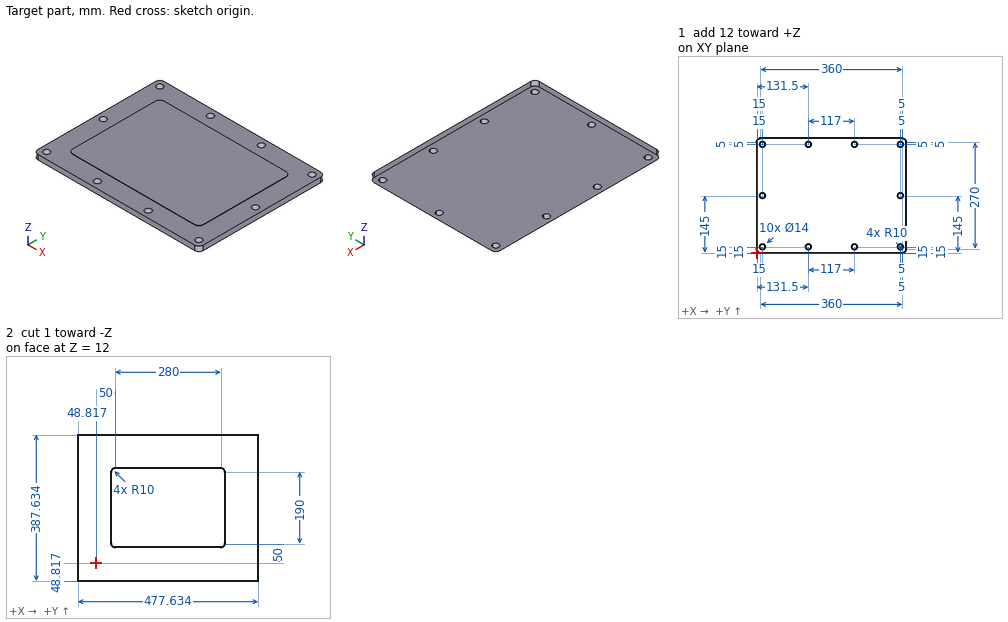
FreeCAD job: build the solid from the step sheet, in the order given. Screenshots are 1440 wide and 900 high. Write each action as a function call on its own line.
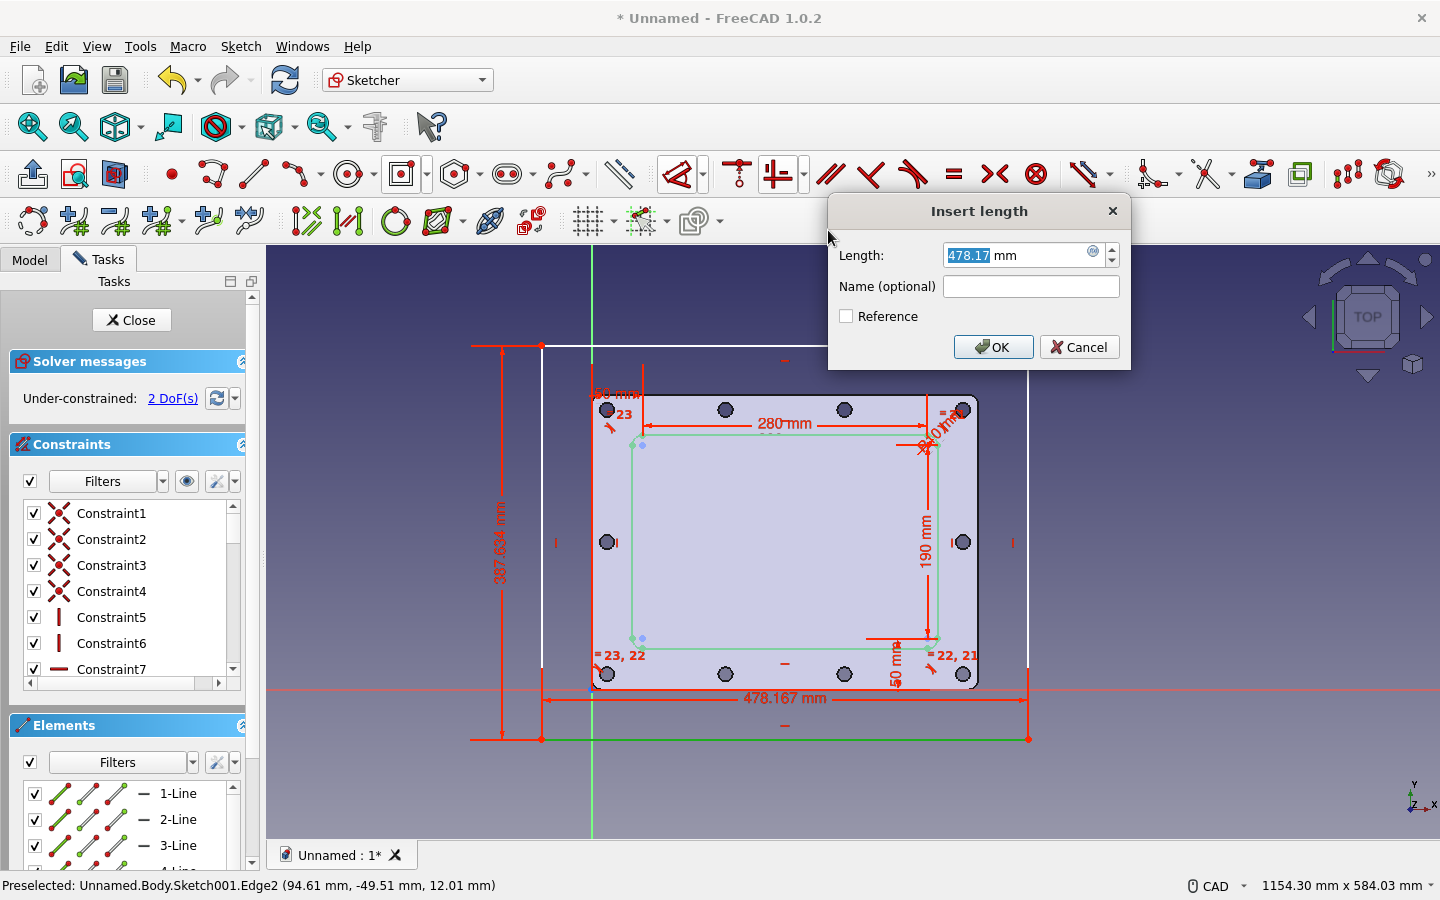
text(477.634)
key(Return)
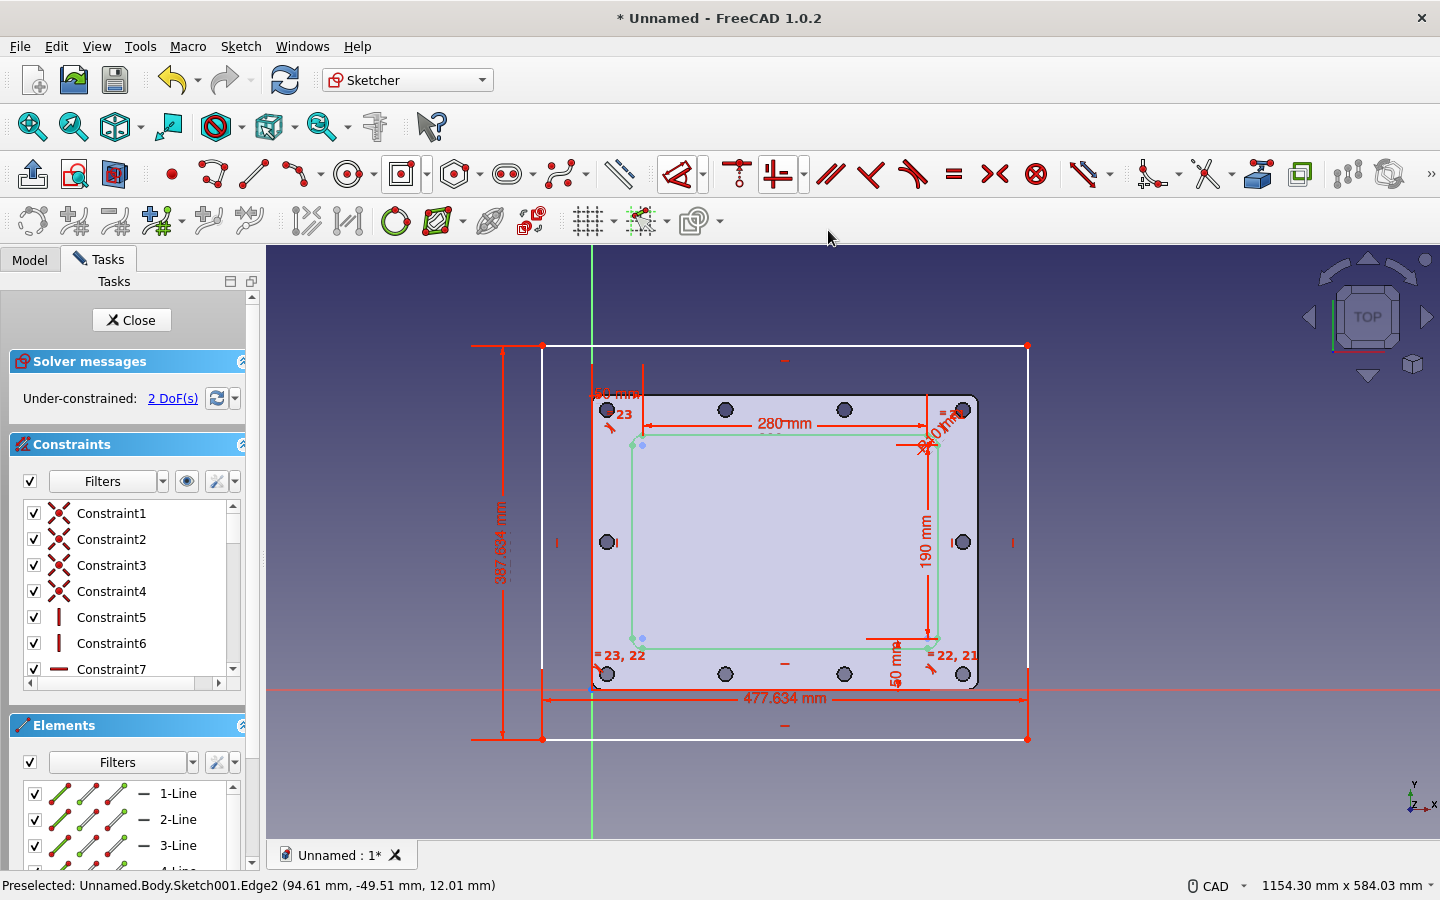
click(542, 346)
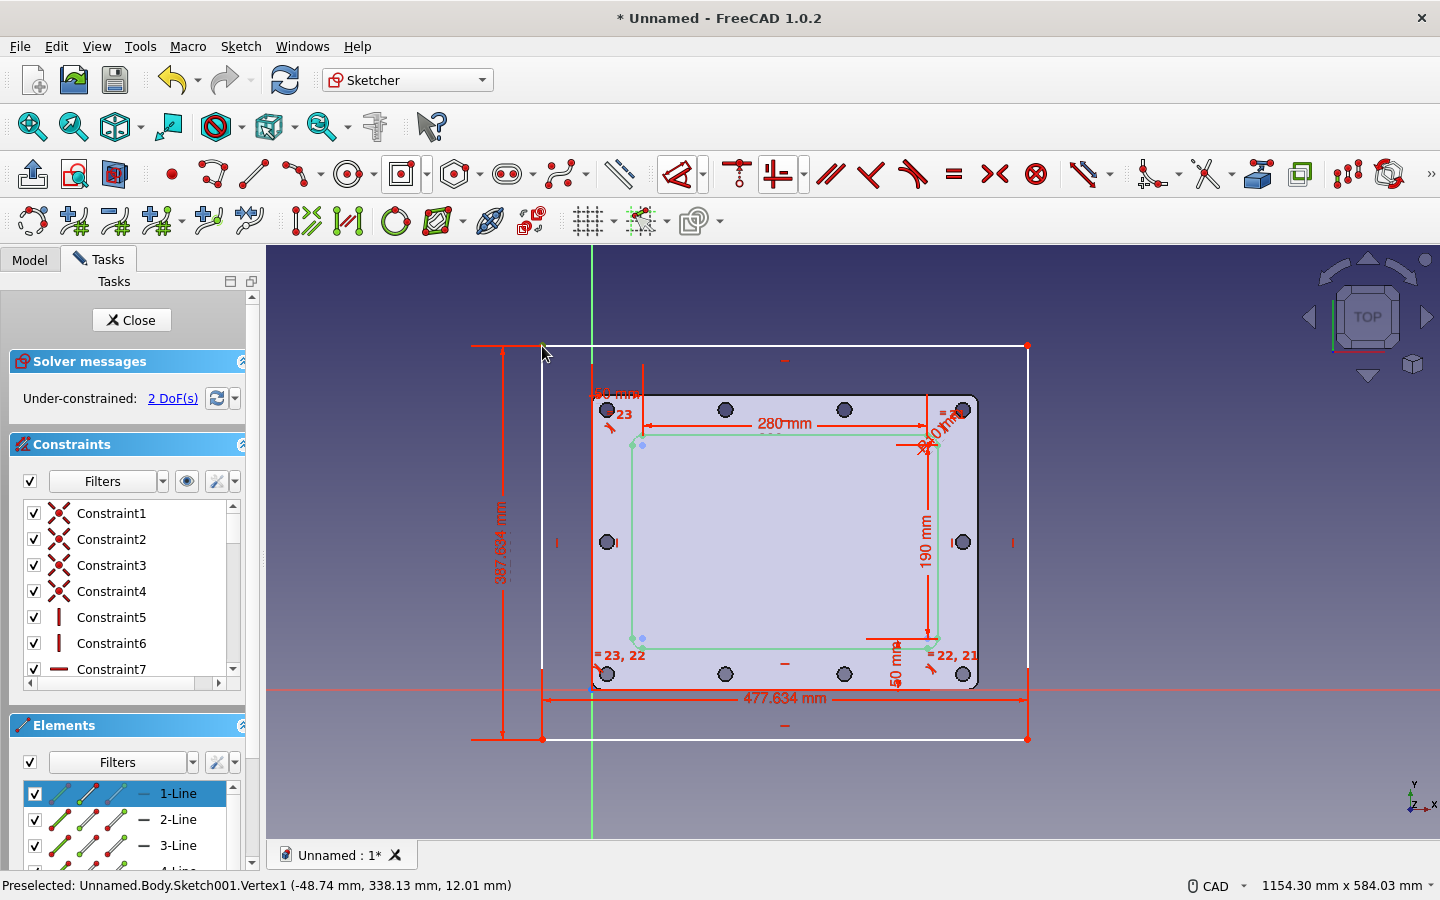
key(l)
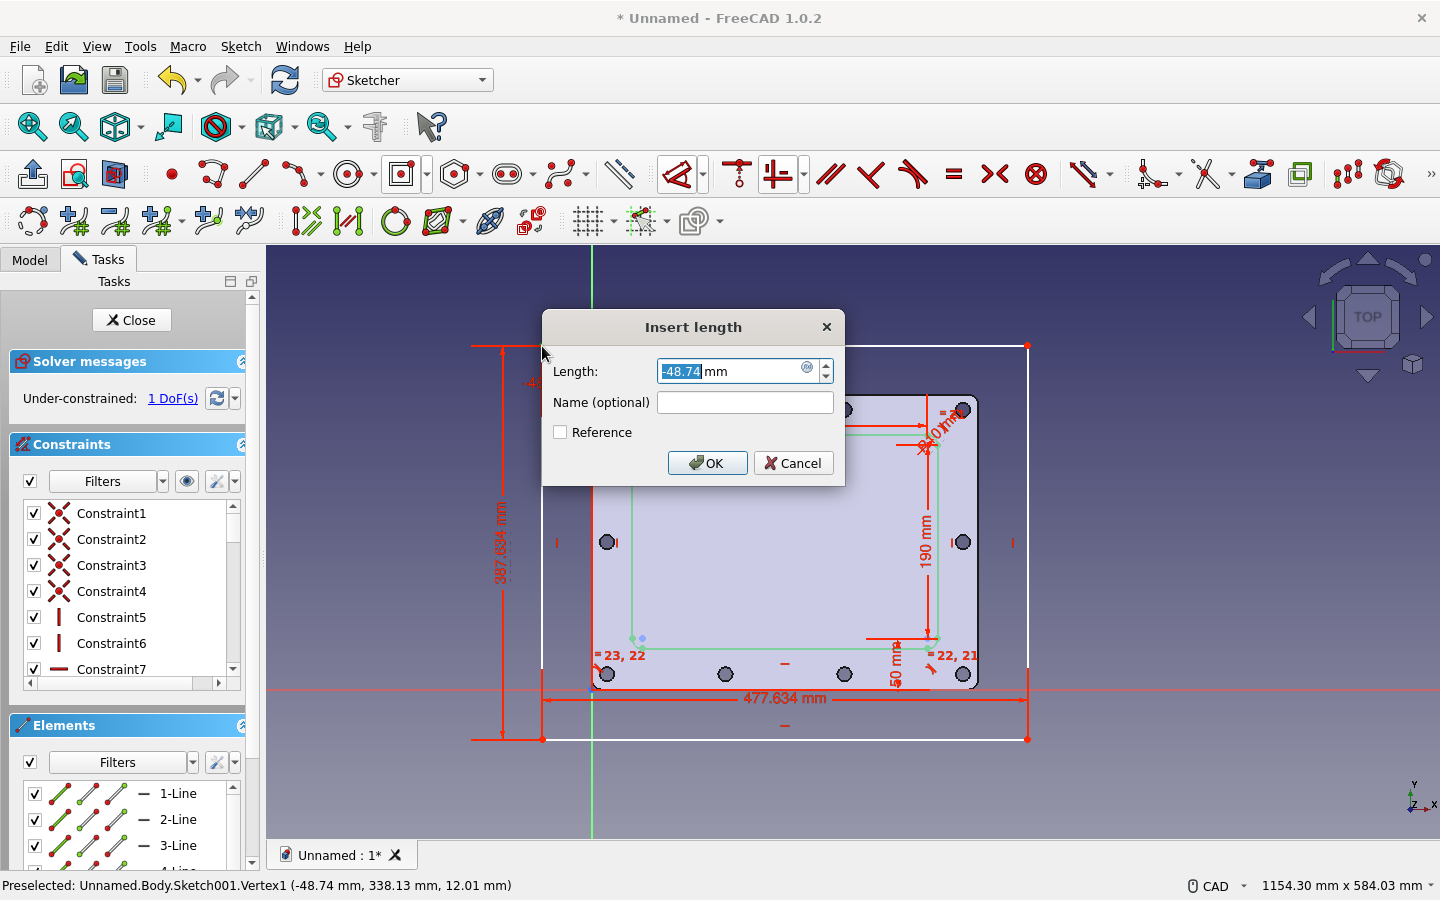
text(-48.817)
key(Return)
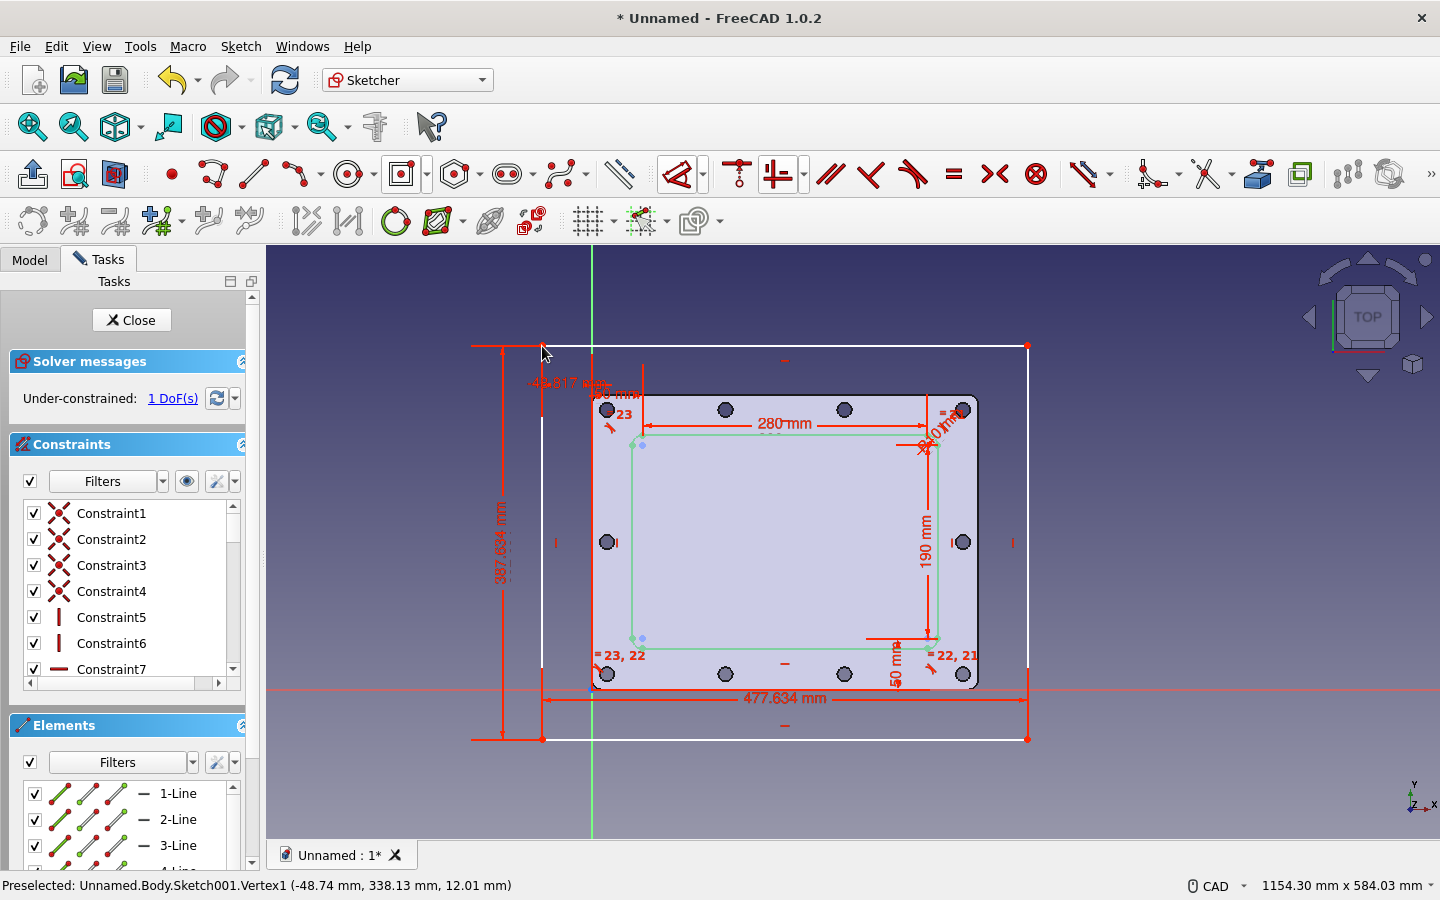
click(542, 740)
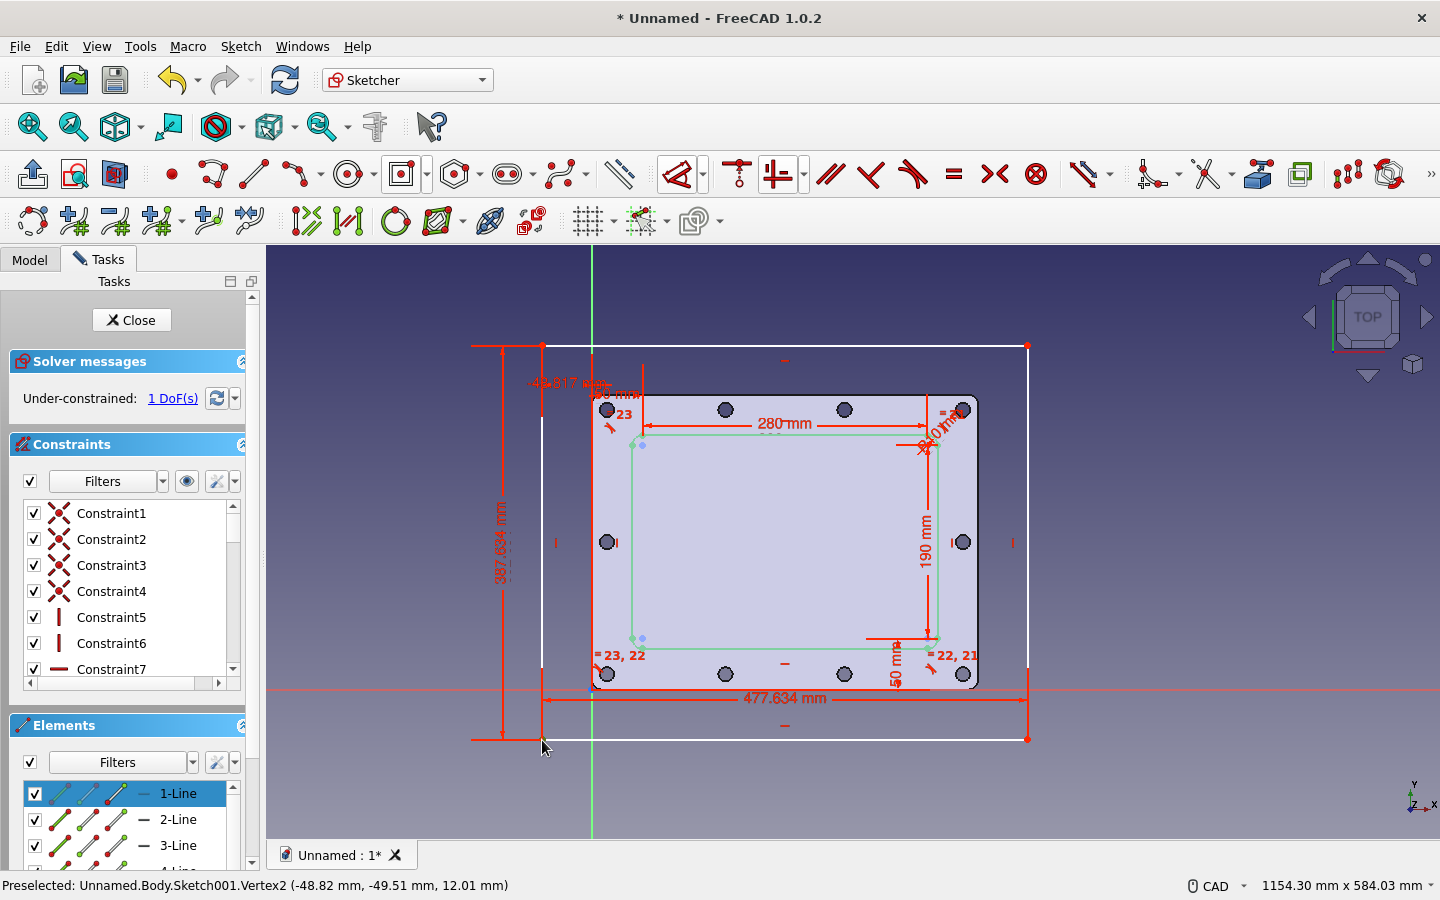
click(702, 174)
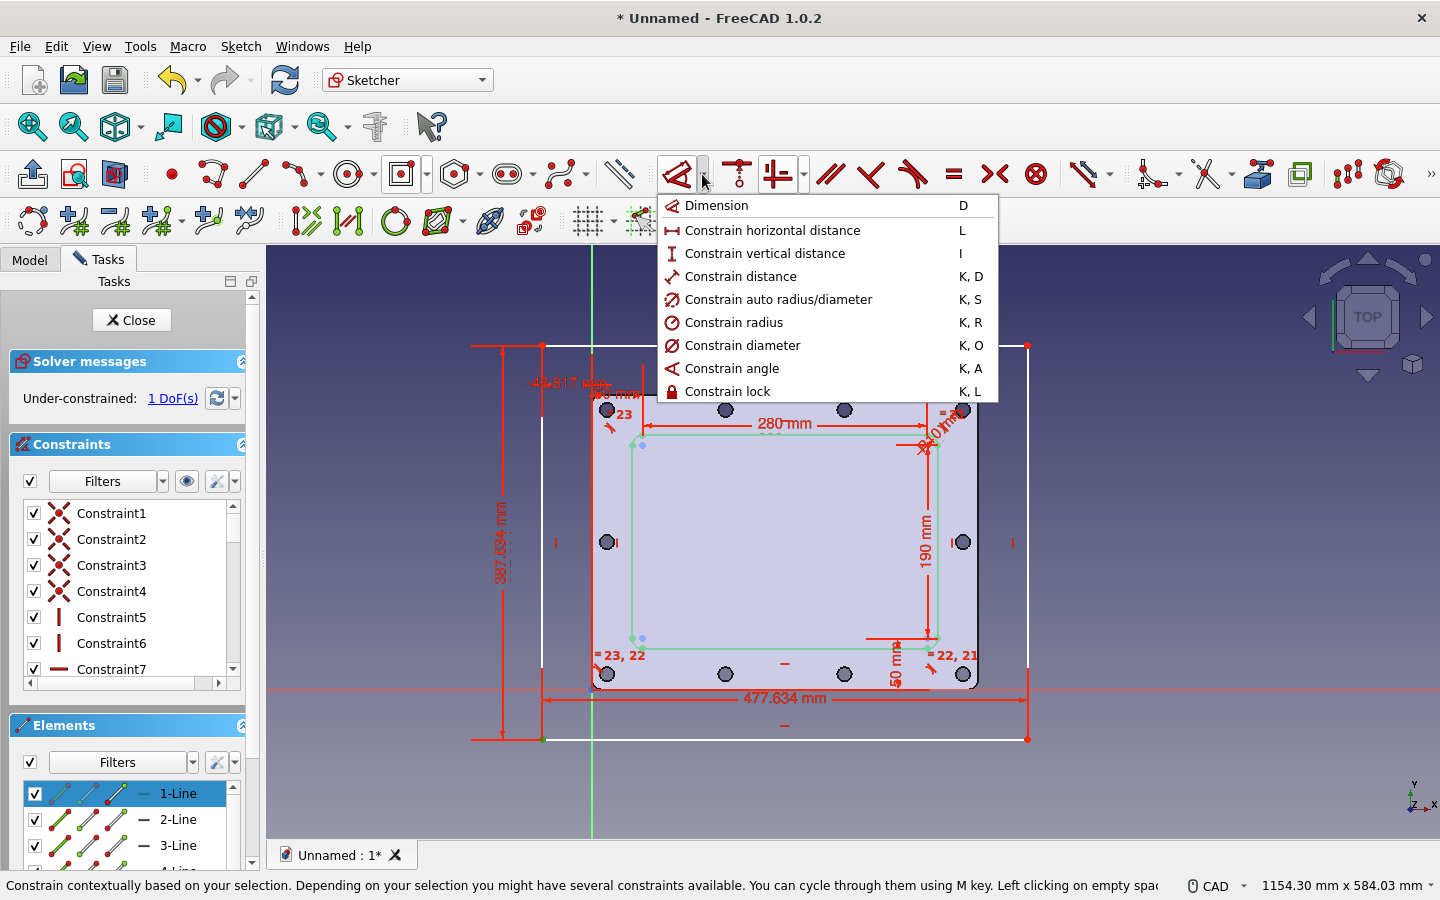
click(828, 254)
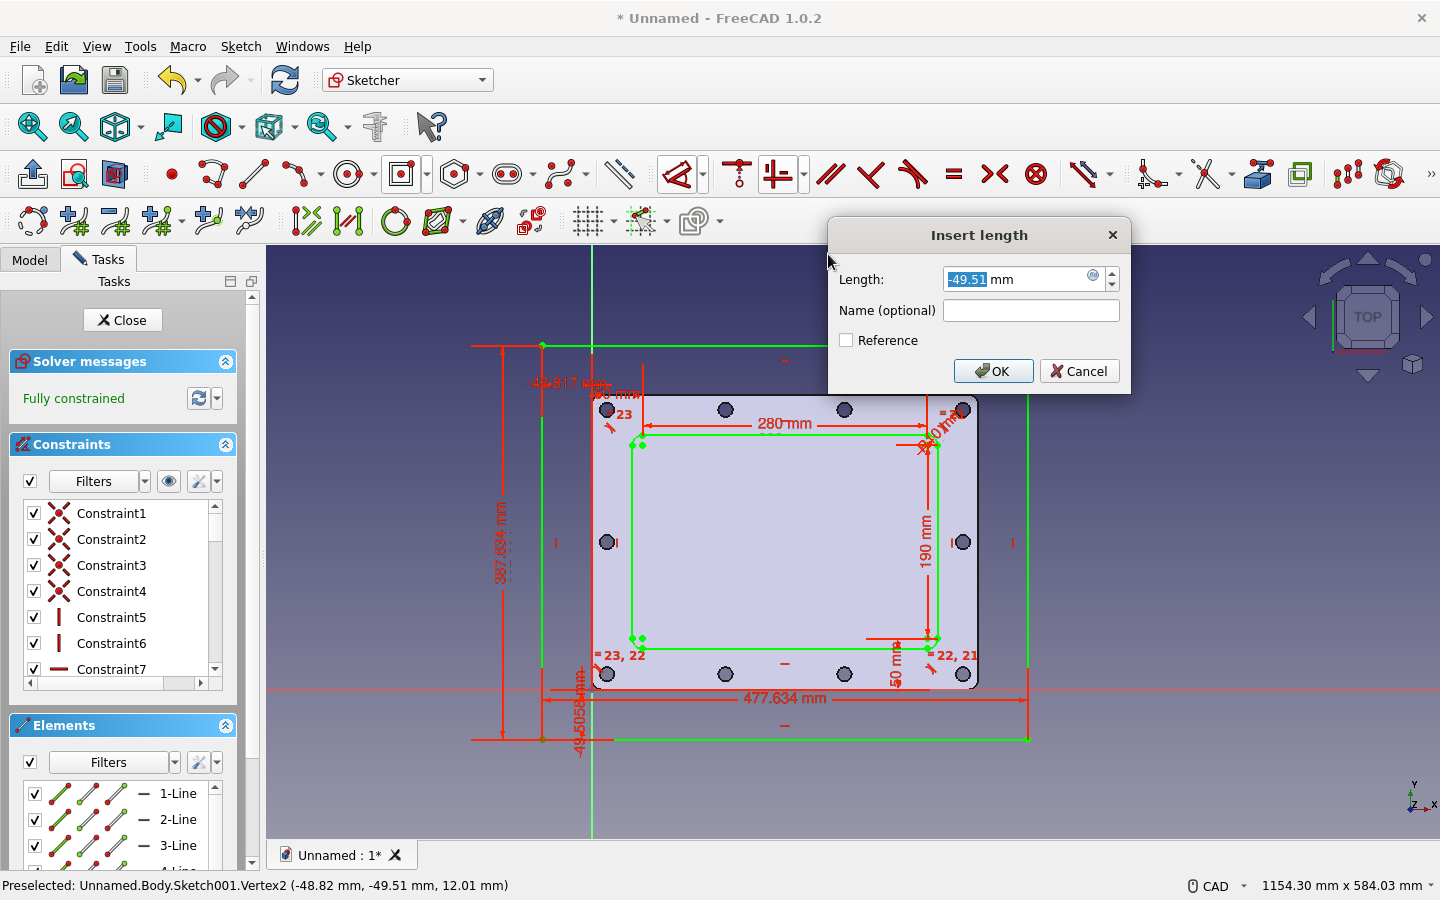
text(-48.817)
key(Return)